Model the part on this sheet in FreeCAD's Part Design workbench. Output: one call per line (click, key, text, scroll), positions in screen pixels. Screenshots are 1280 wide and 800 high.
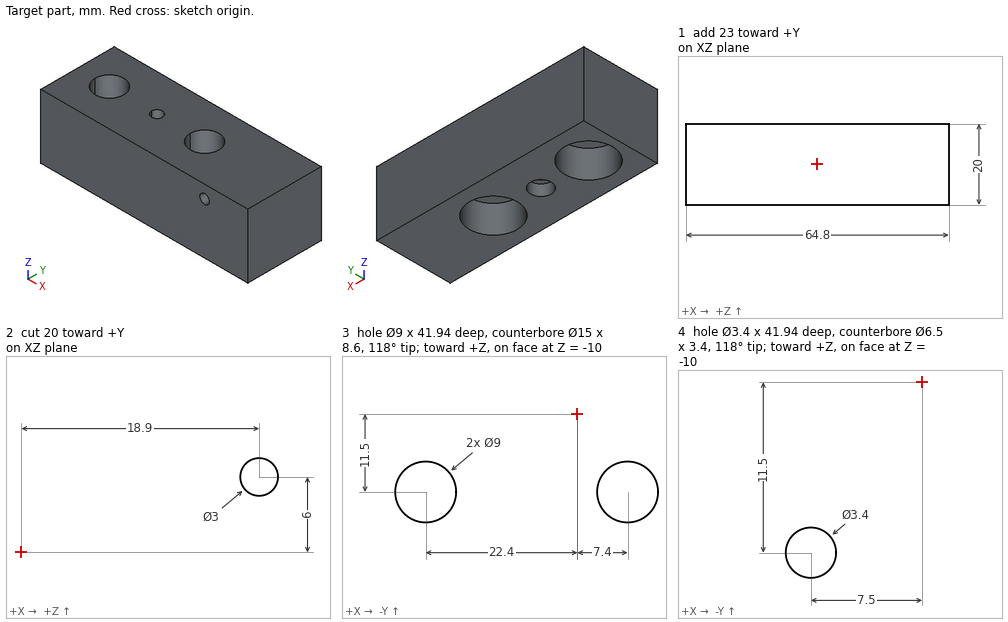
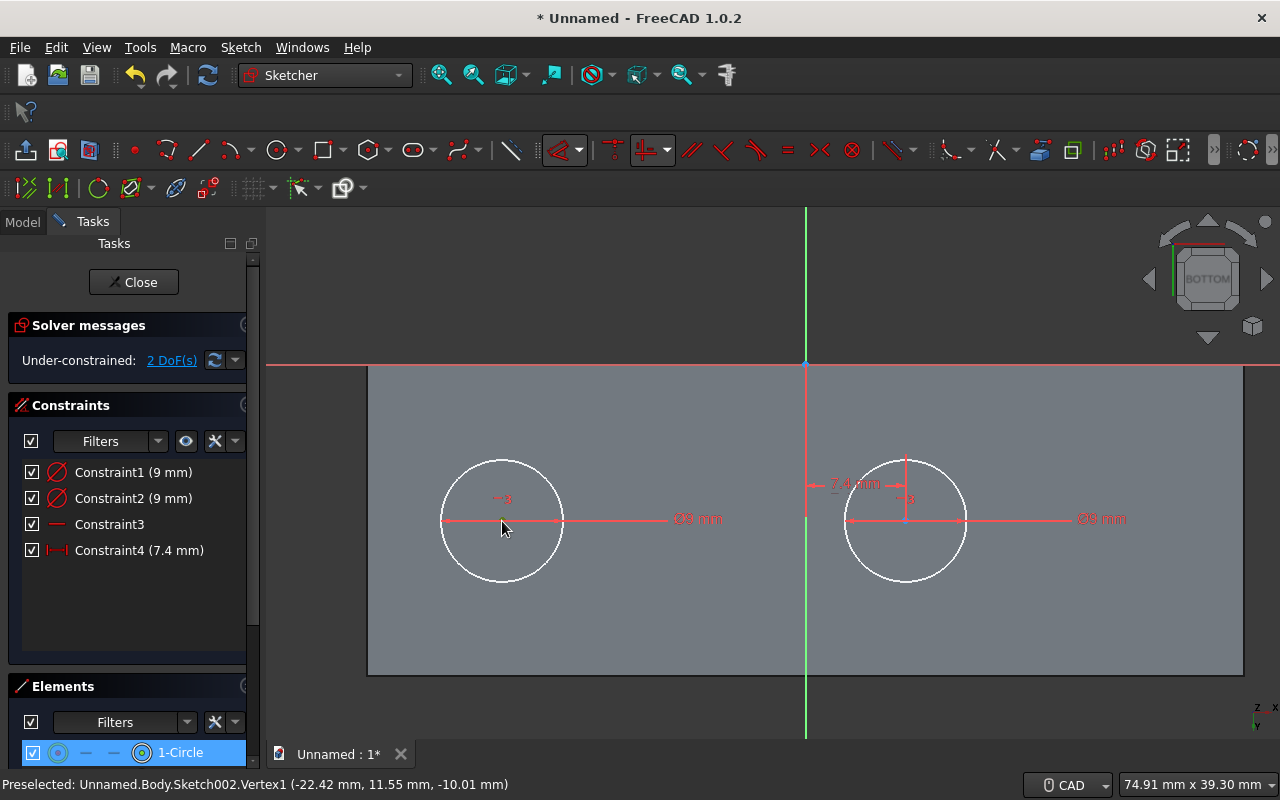
key(l)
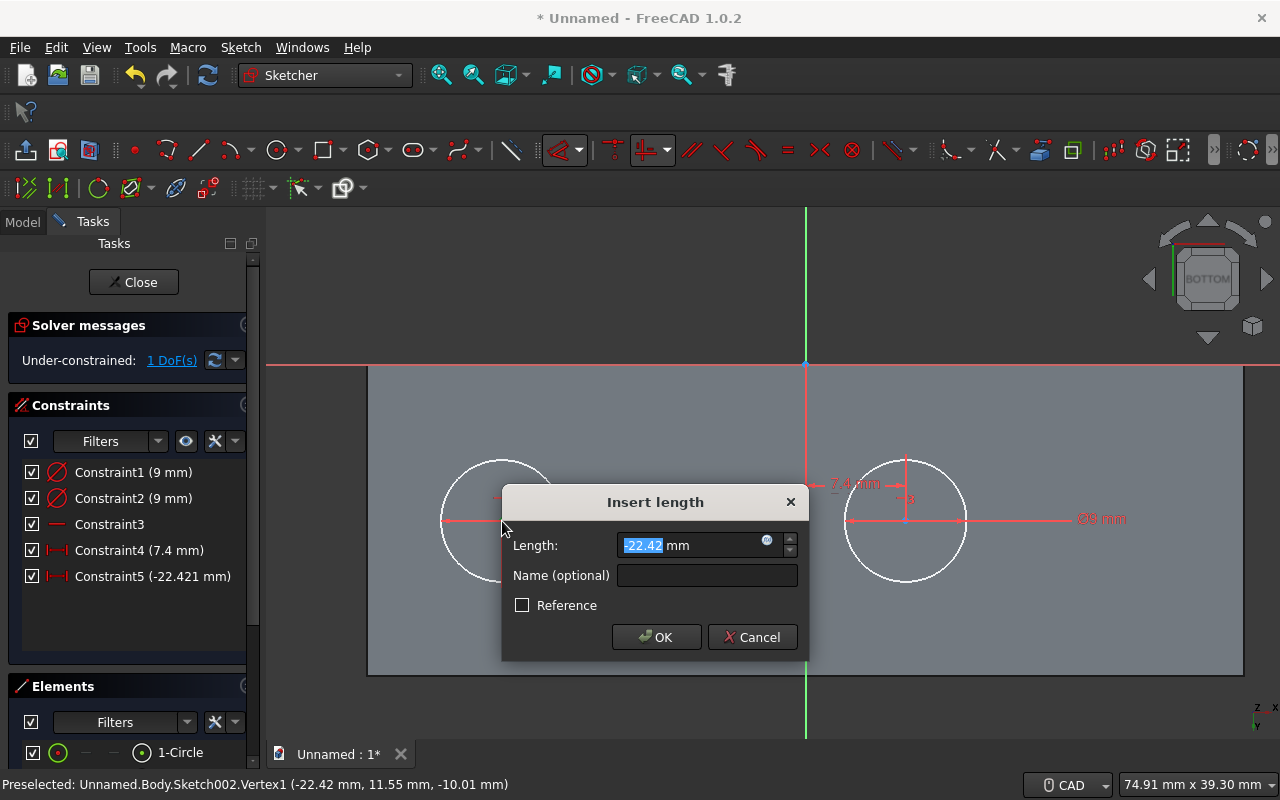
text(-22.4)
key(Return)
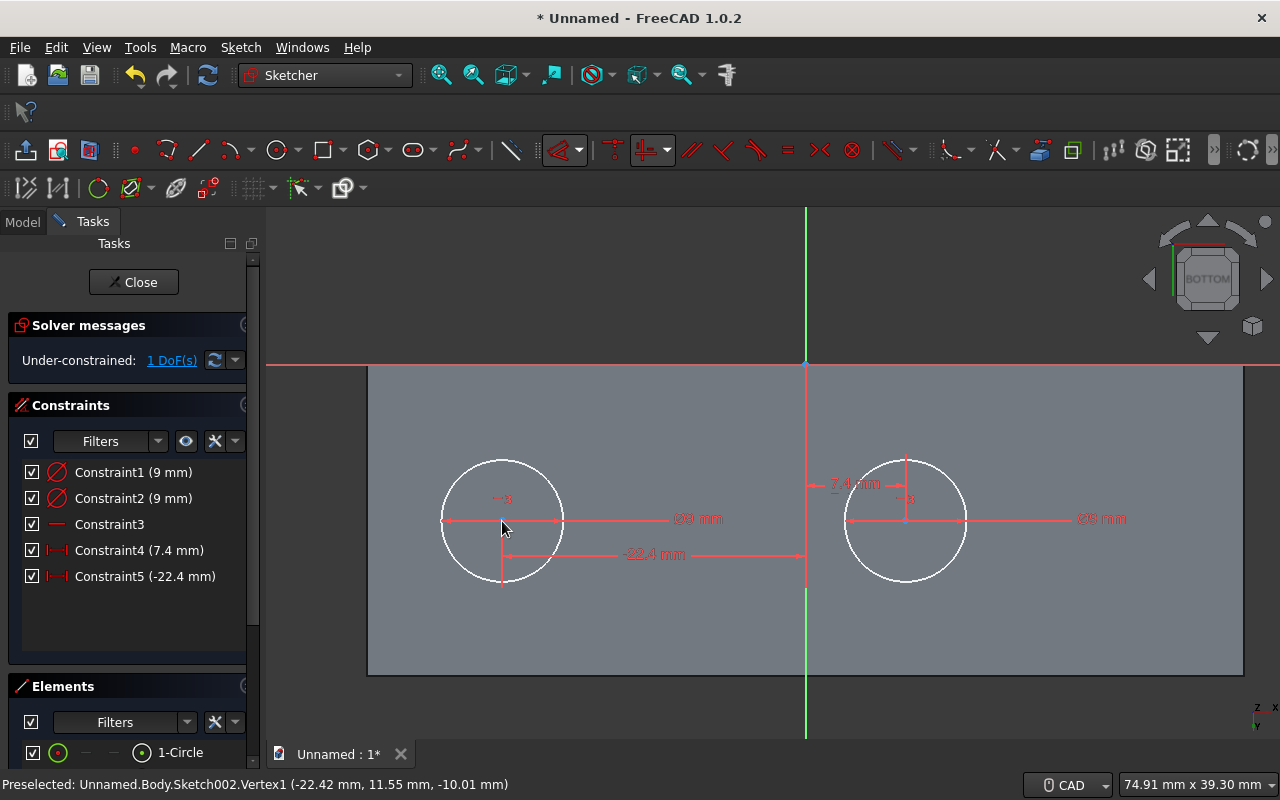
click(502, 521)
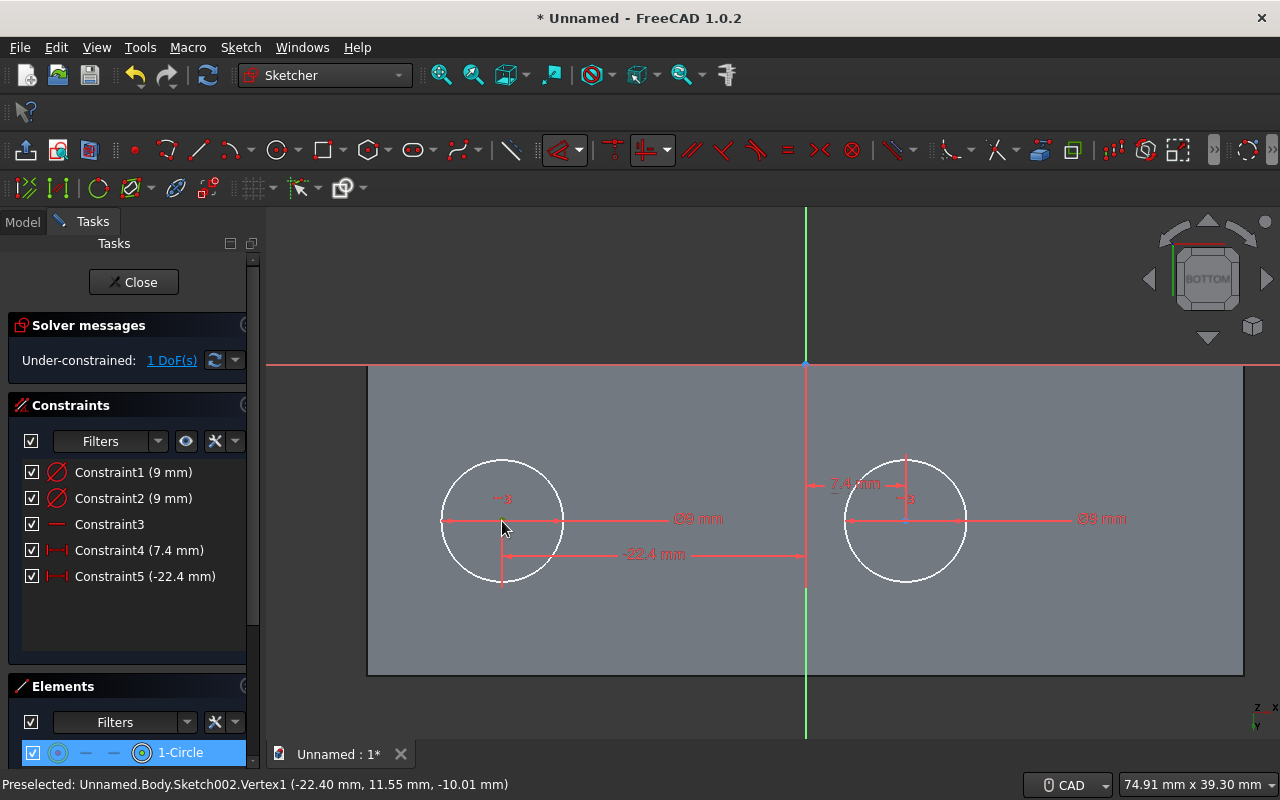
key(i)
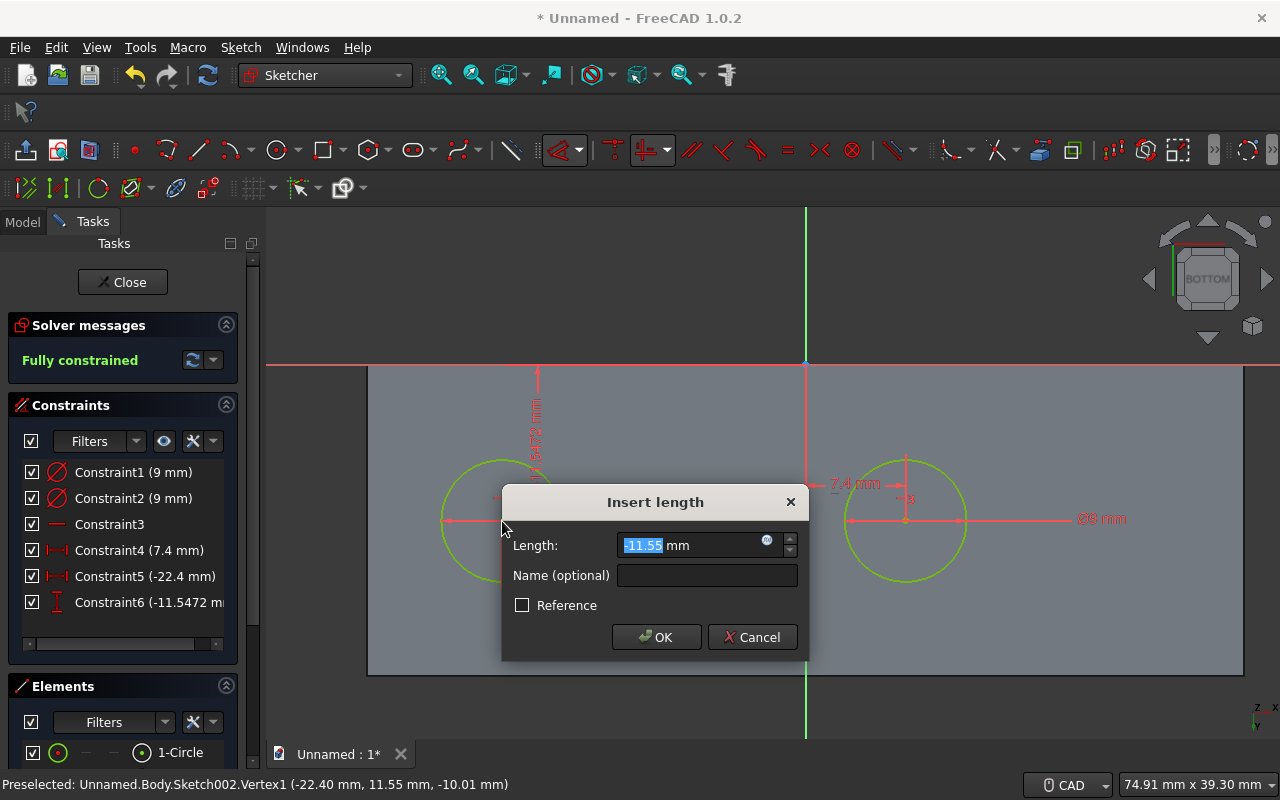
text(-11.5)
key(Return)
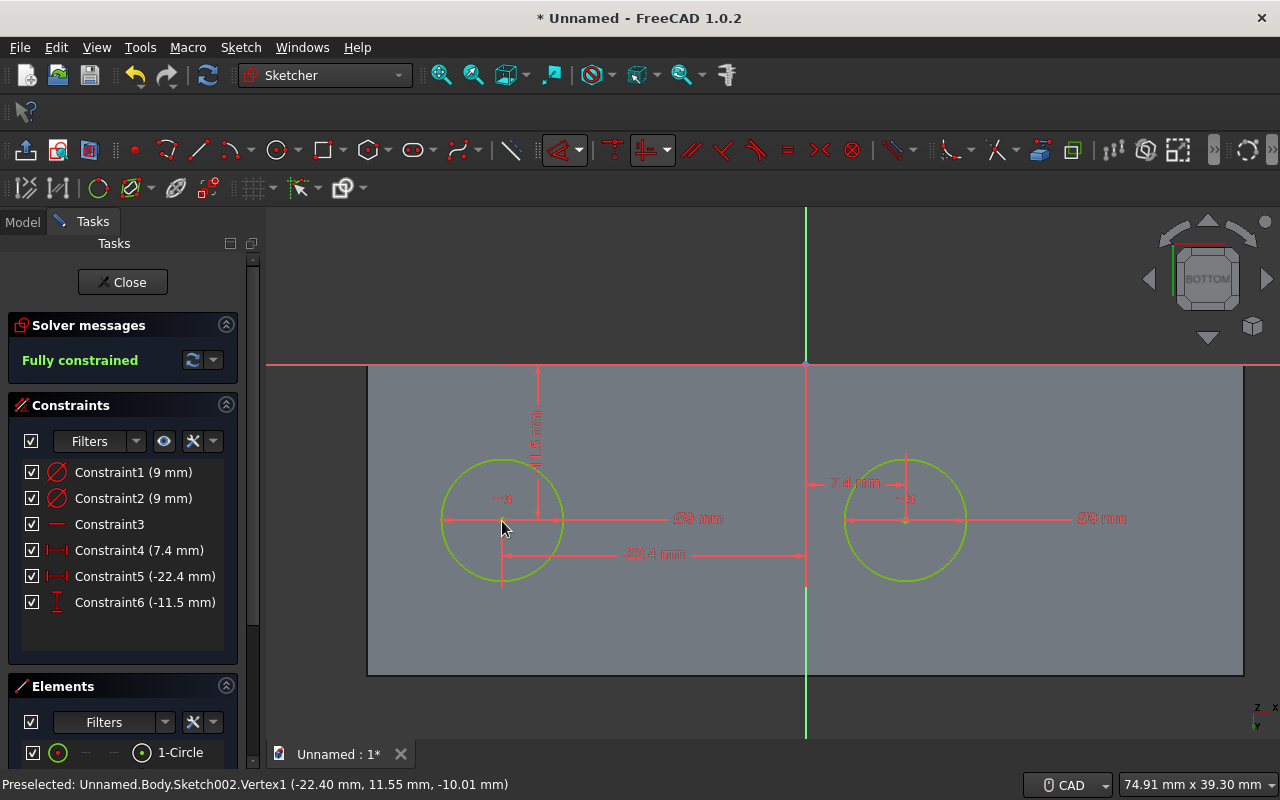
click(123, 282)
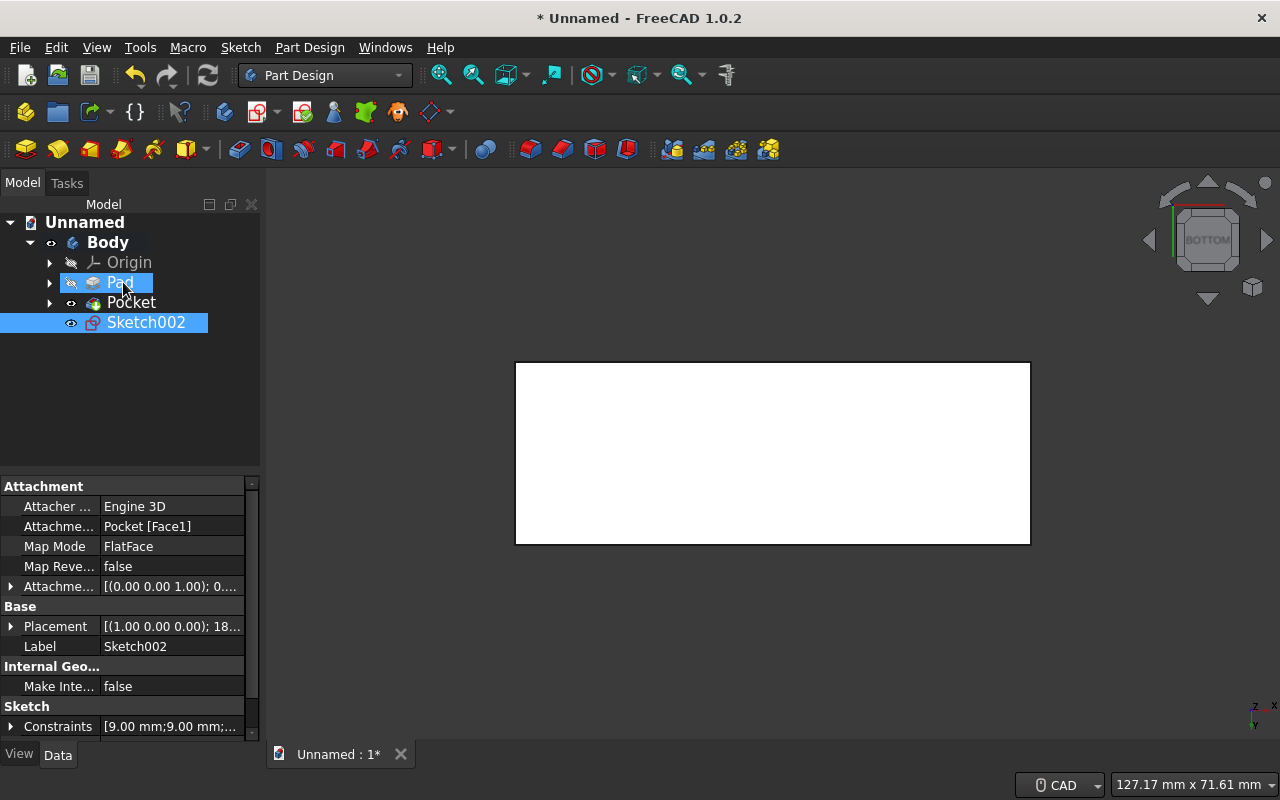
click(272, 150)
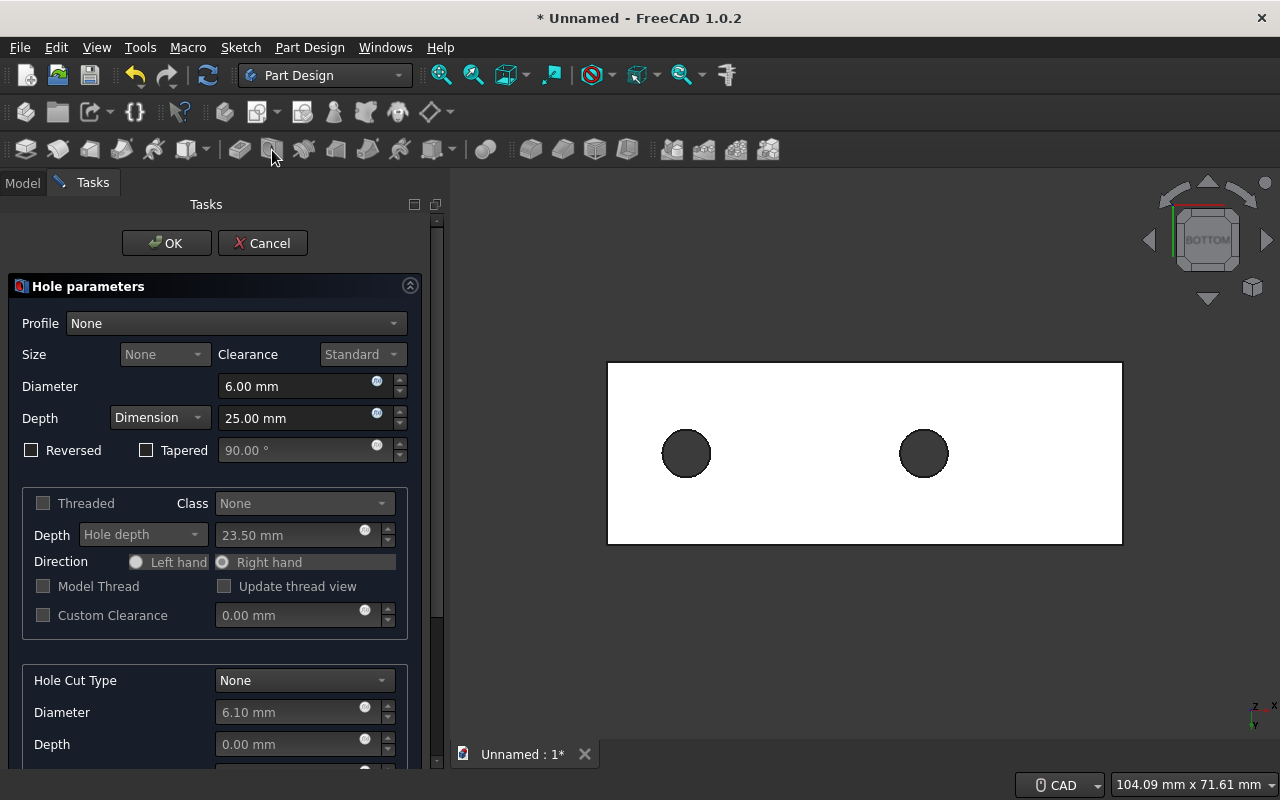
triple_click(305, 386)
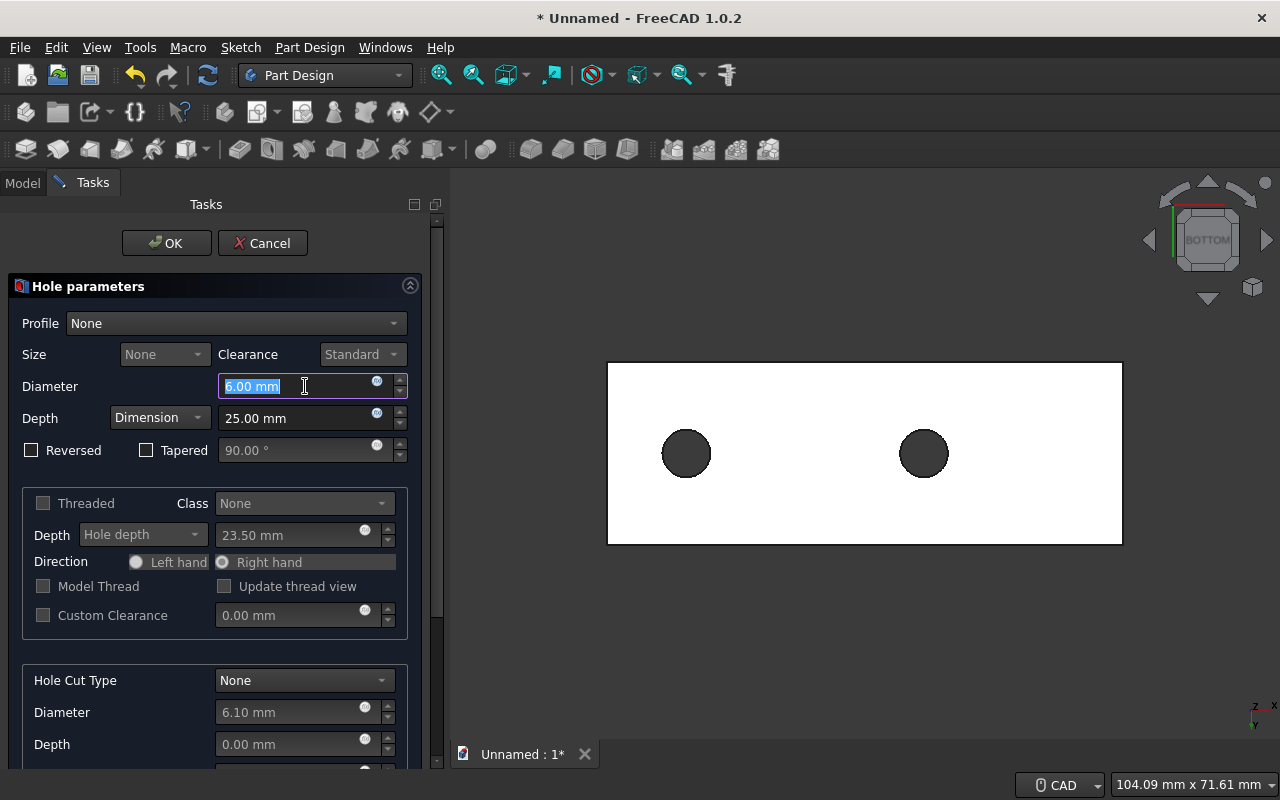
text(9)
key(Tab)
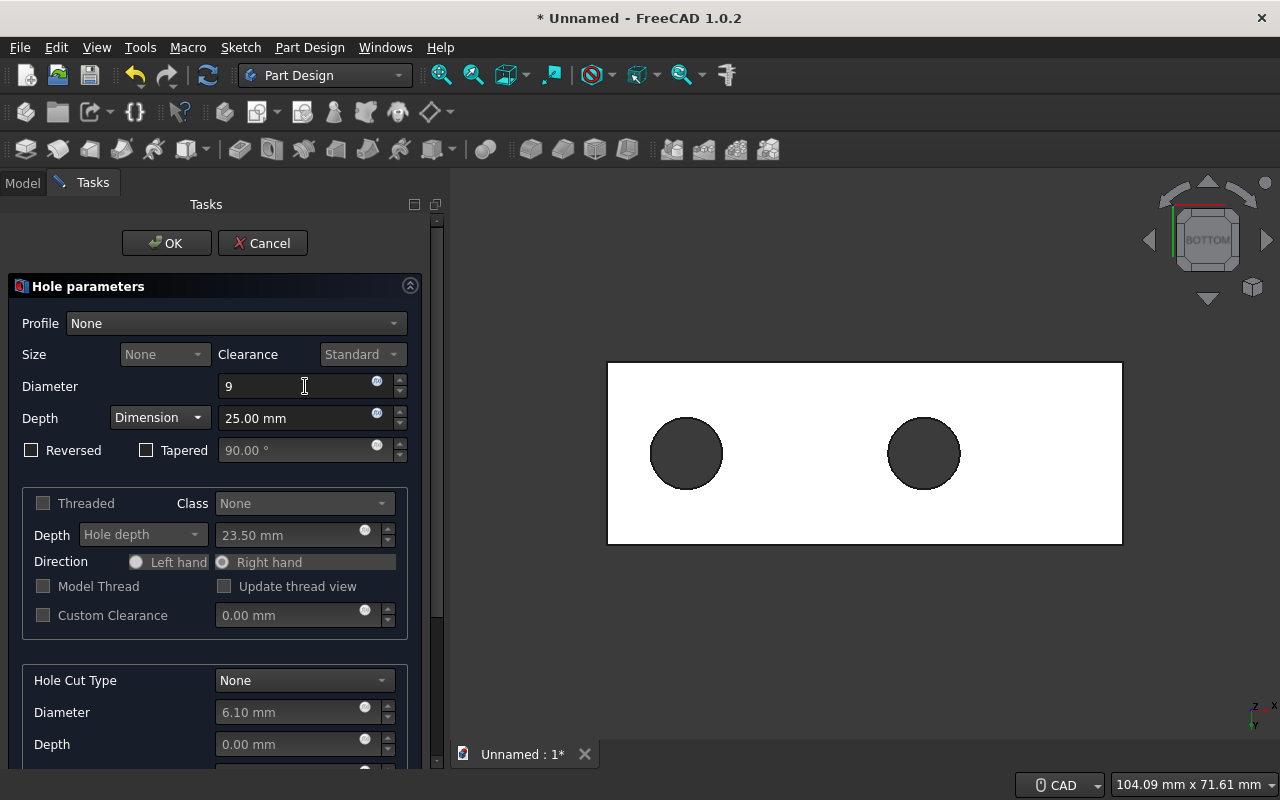
triple_click(305, 418)